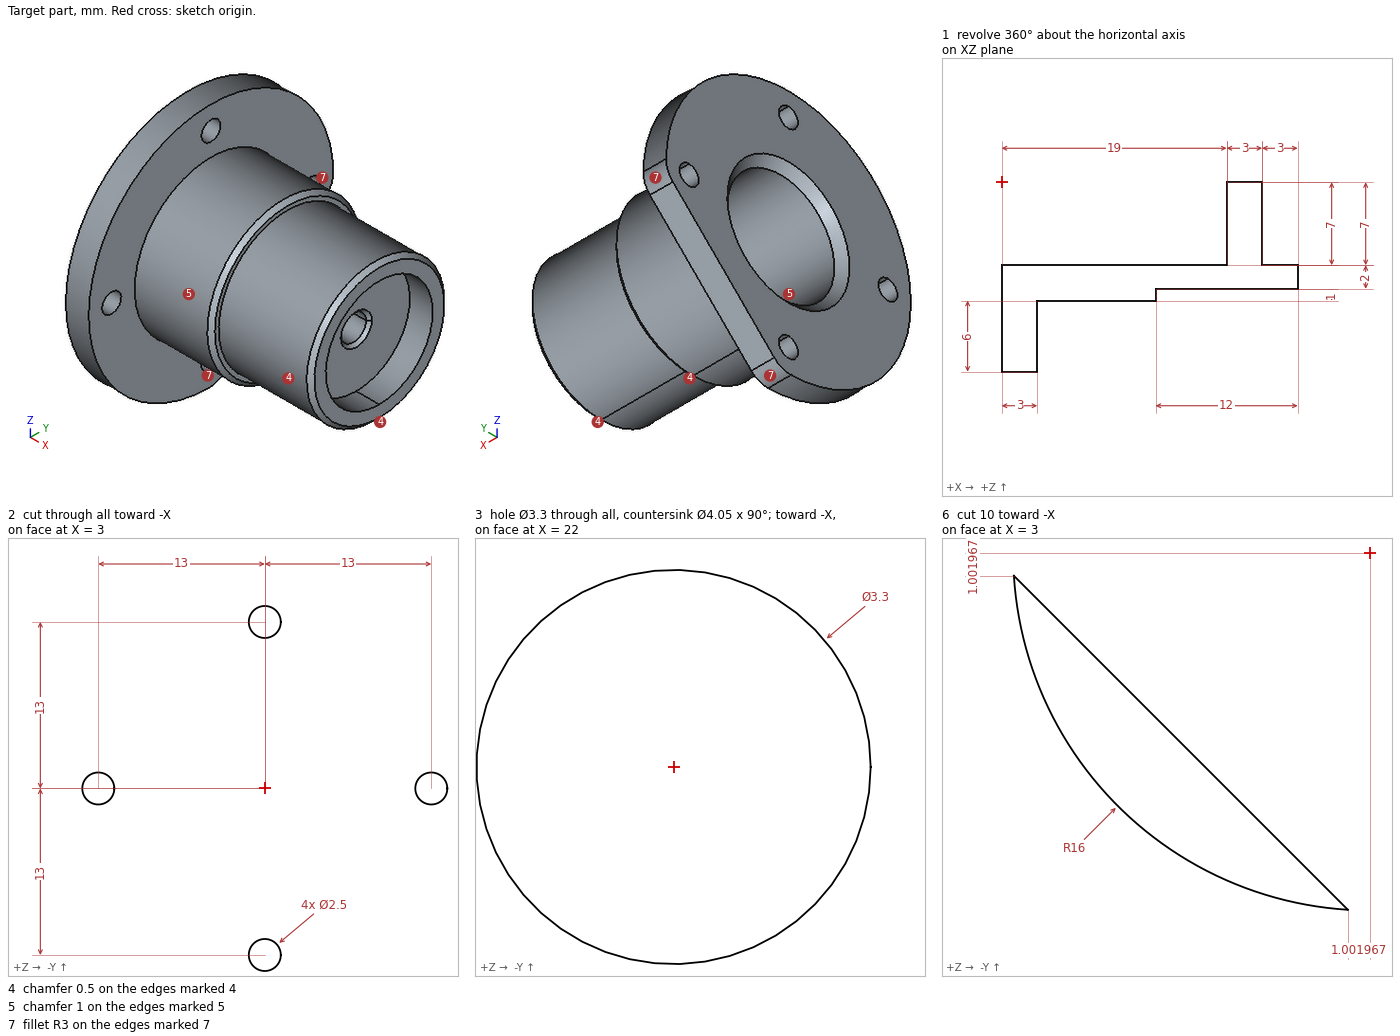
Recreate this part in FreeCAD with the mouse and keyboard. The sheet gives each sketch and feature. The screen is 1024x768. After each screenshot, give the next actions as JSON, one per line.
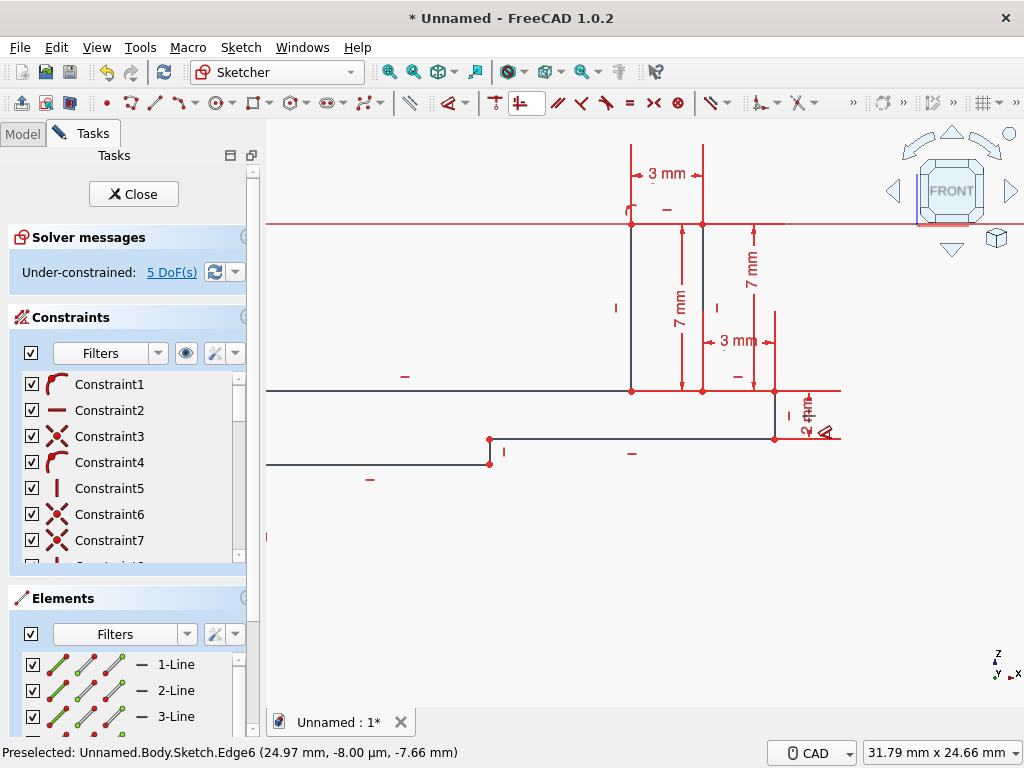
{"action": "scroll", "coordinate": [490, 449], "scroll_direction": "up", "scroll_amount": 3}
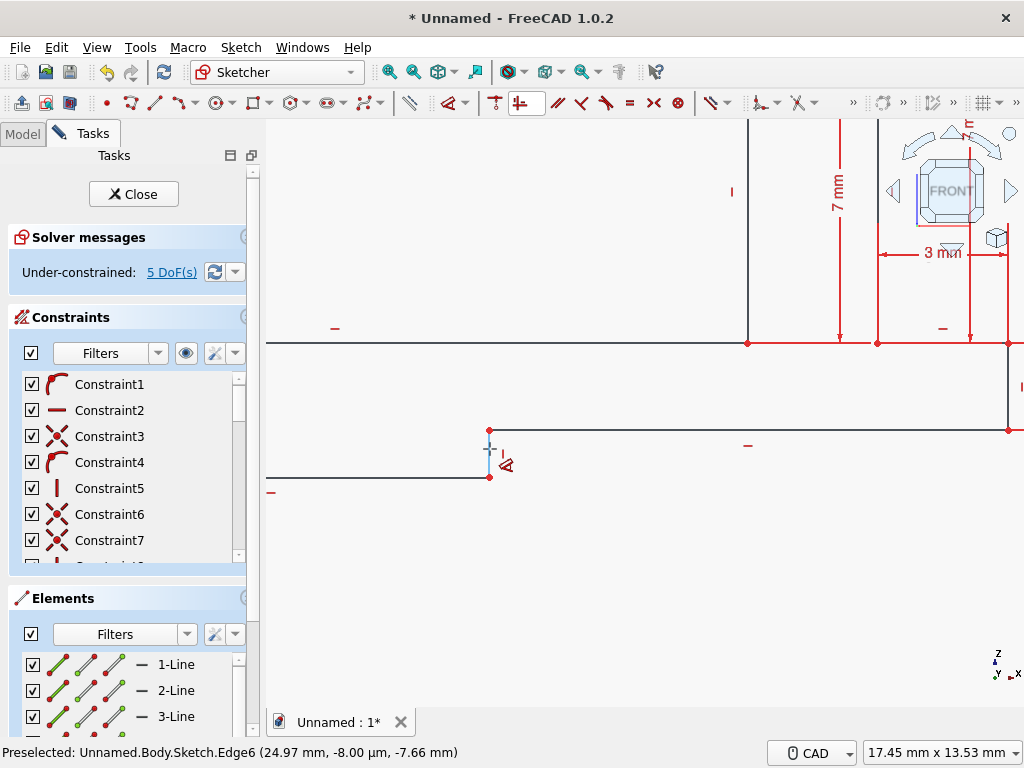
{"action": "left_click", "coordinate": [489, 449]}
{"action": "left_click", "coordinate": [523, 454]}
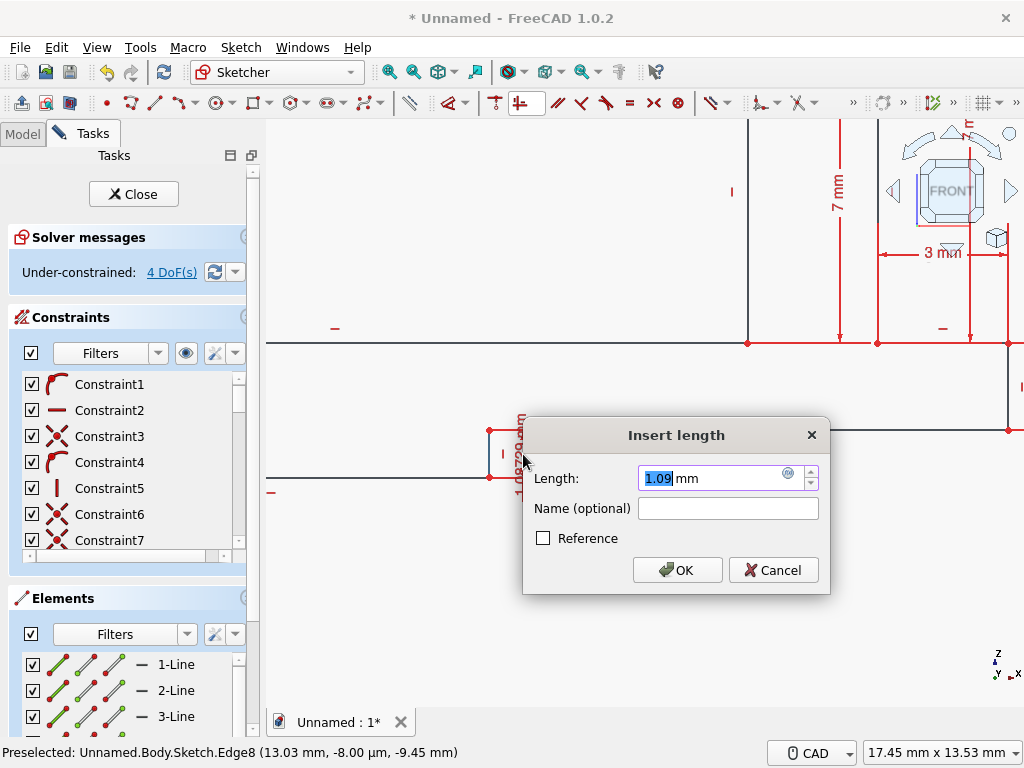
{"action": "type", "text": "1"}
{"action": "key", "text": "Return"}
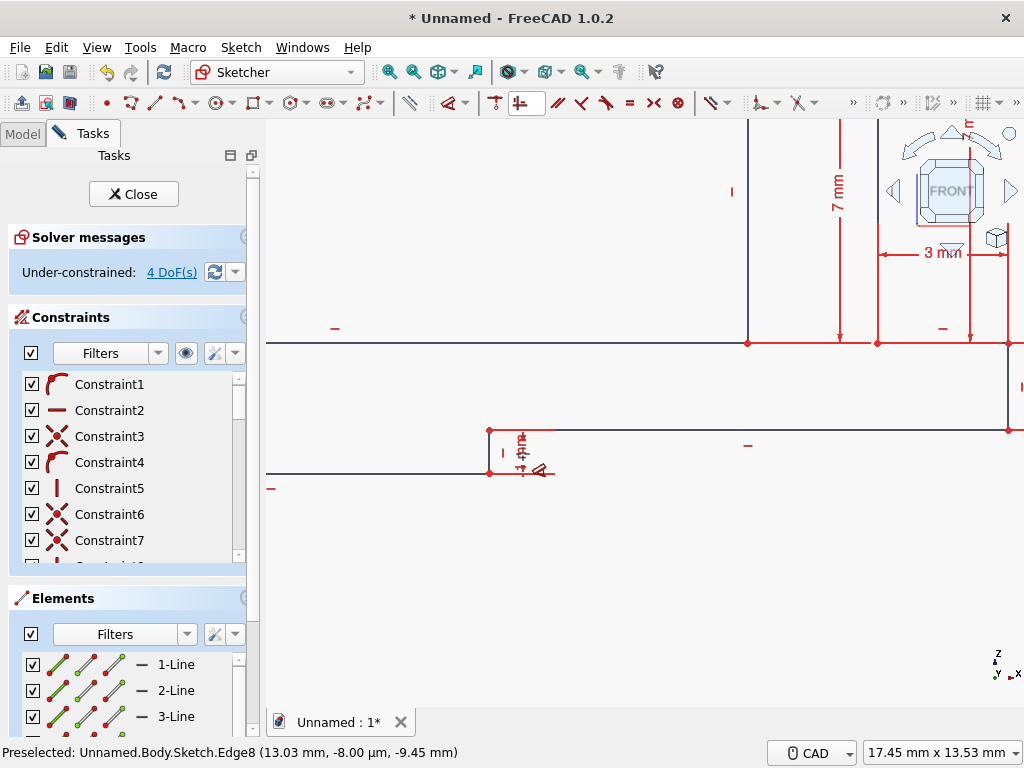
{"action": "scroll", "coordinate": [641, 428], "scroll_direction": "down", "scroll_amount": 5}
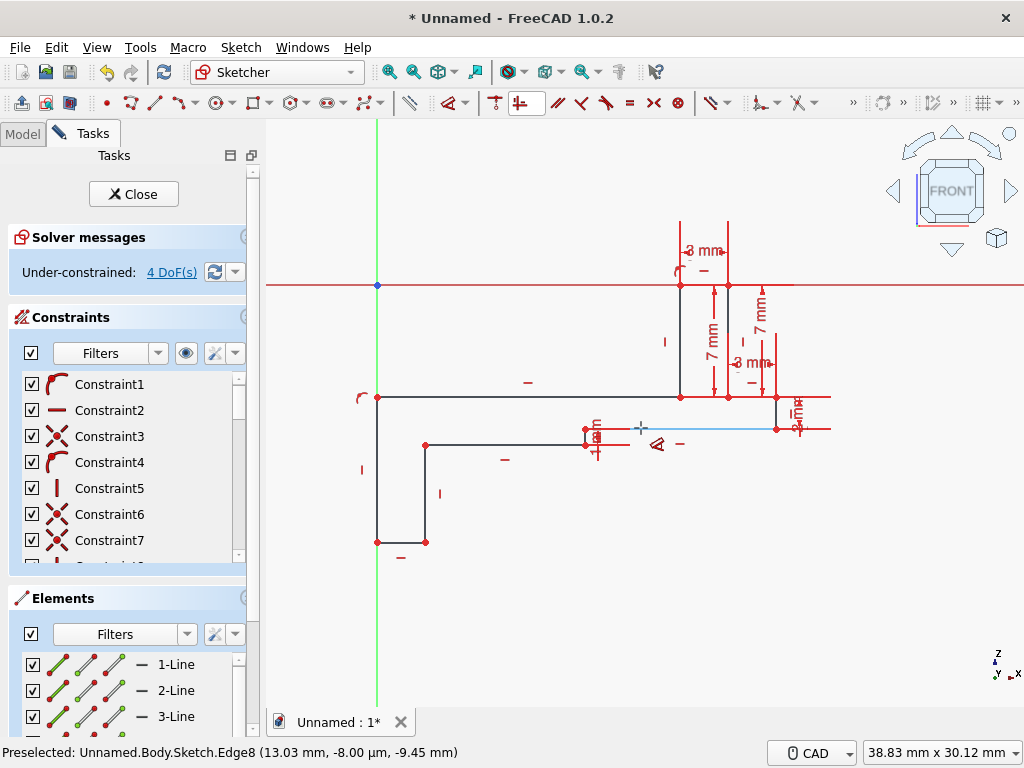
{"action": "left_click", "coordinate": [425, 474]}
{"action": "left_click", "coordinate": [391, 494]}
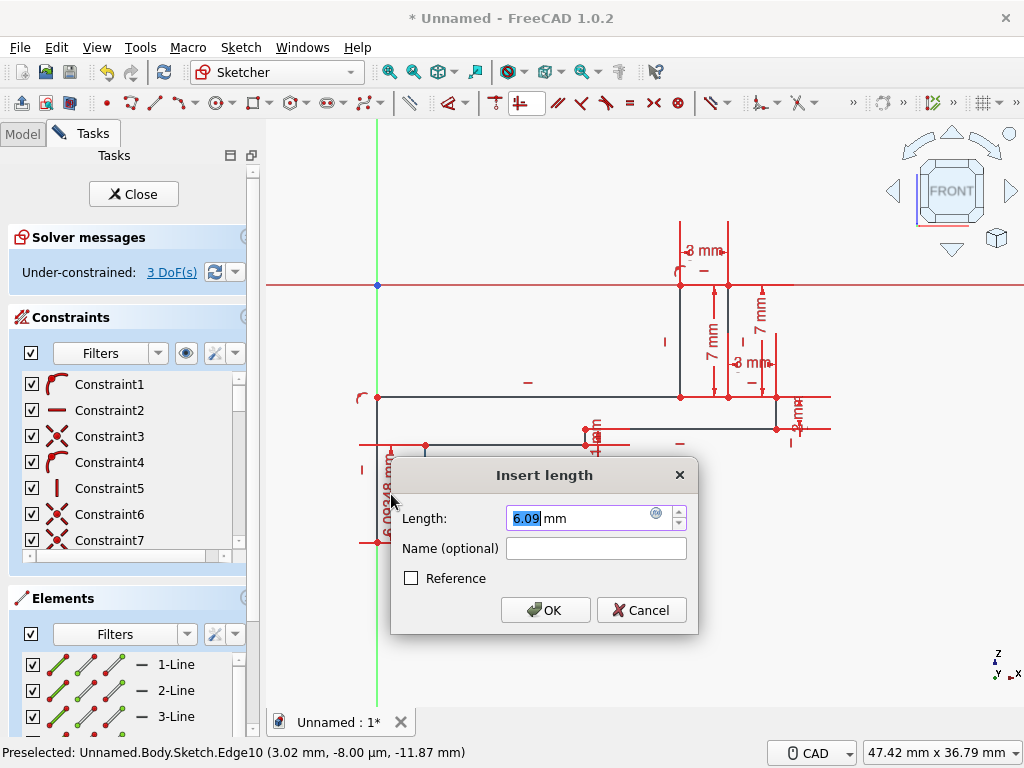
{"action": "type", "text": "6"}
{"action": "key", "text": "Return"}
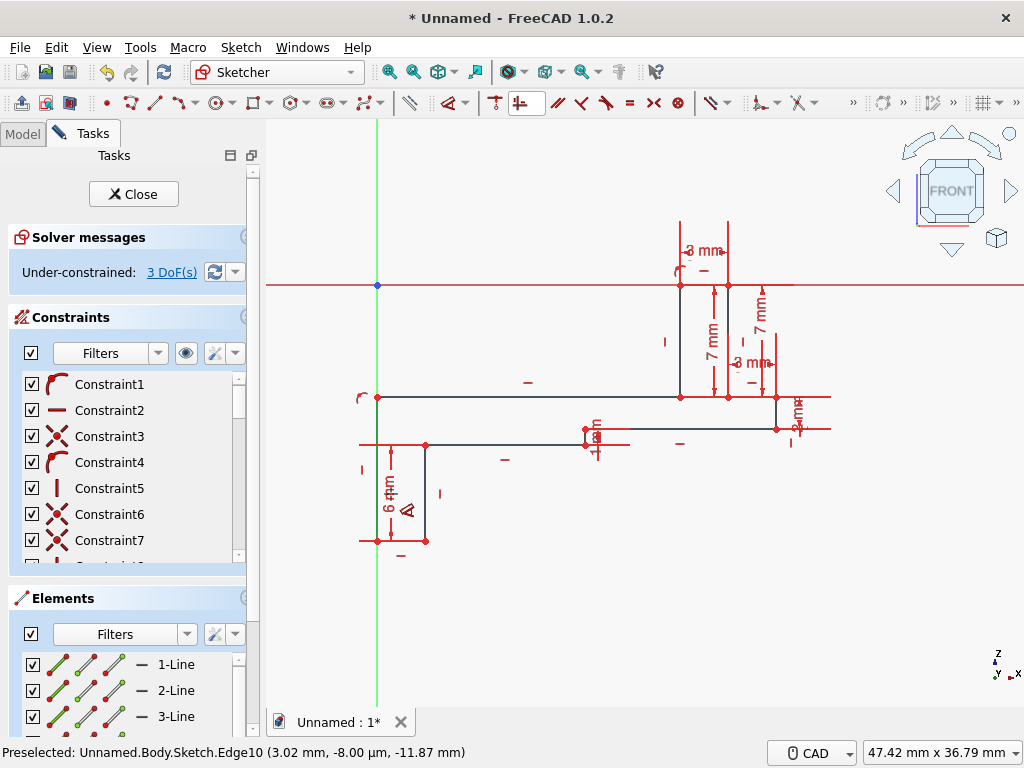
{"action": "left_click", "coordinate": [411, 541]}
{"action": "left_click", "coordinate": [401, 575]}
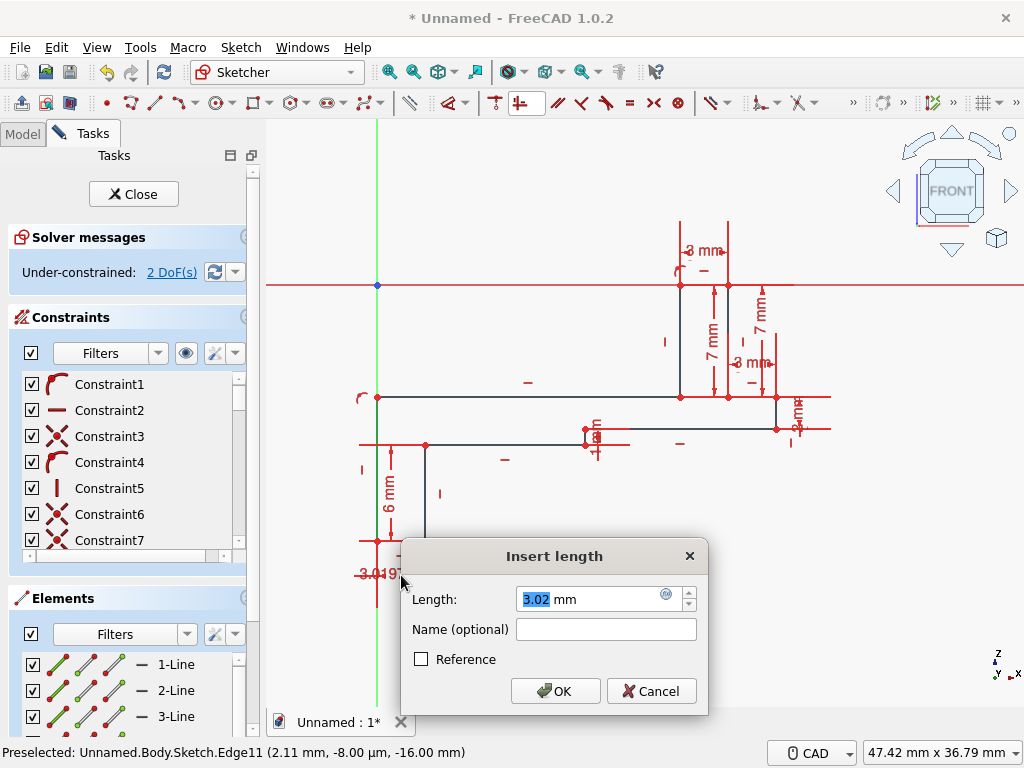
{"action": "type", "text": "3"}
{"action": "key", "text": "Return"}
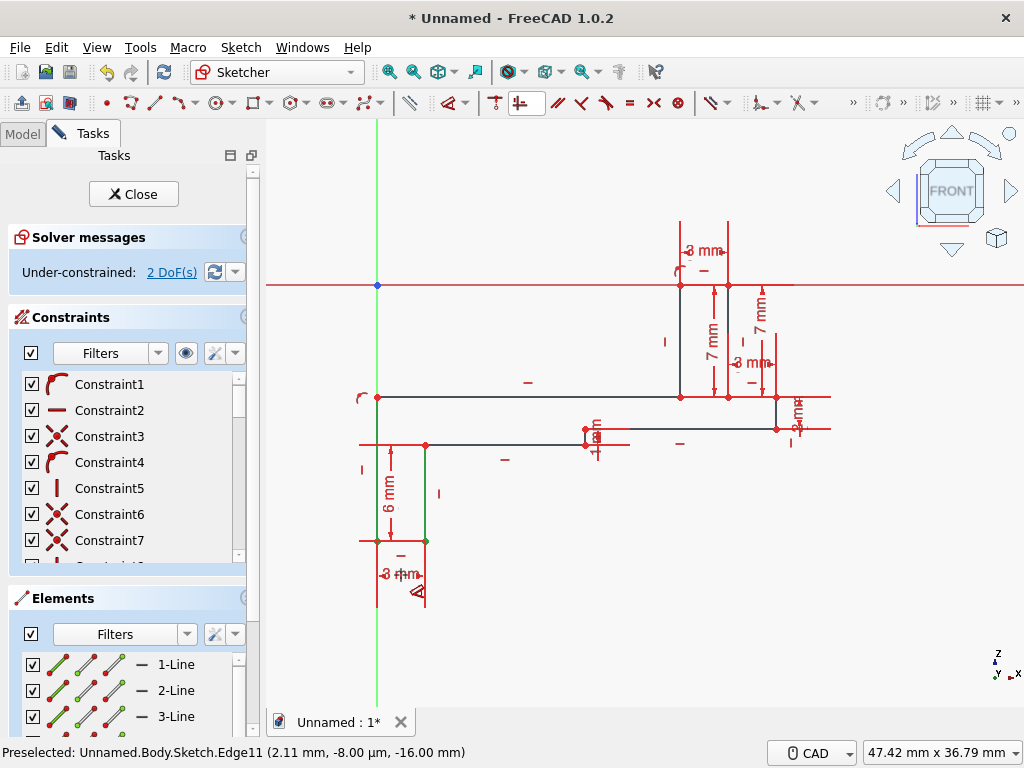
{"action": "left_click", "coordinate": [468, 397]}
{"action": "left_click", "coordinate": [529, 363]}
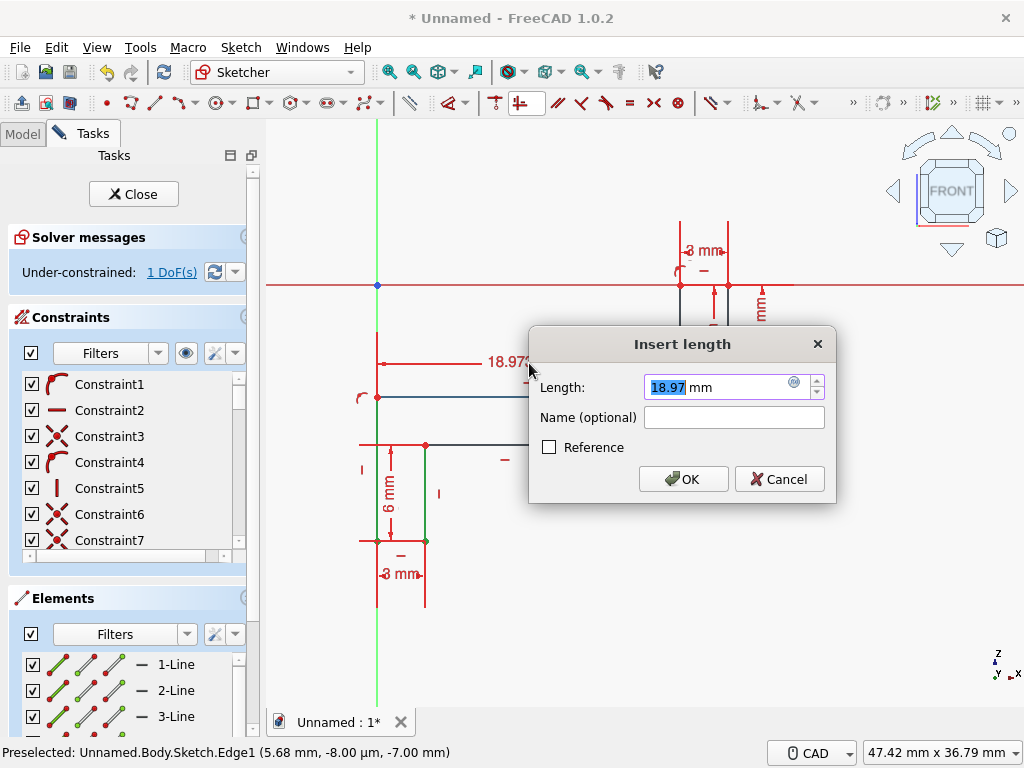
{"action": "type", "text": "19"}
{"action": "key", "text": "Return"}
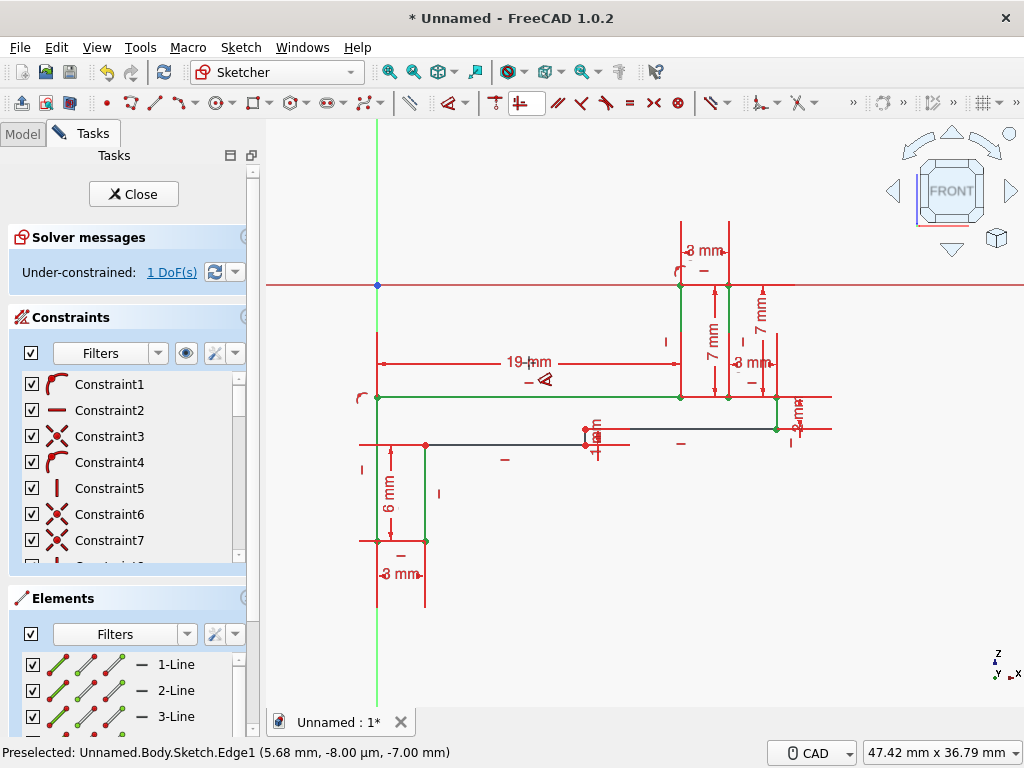
{"action": "left_click", "coordinate": [719, 429]}
{"action": "left_click", "coordinate": [681, 463]}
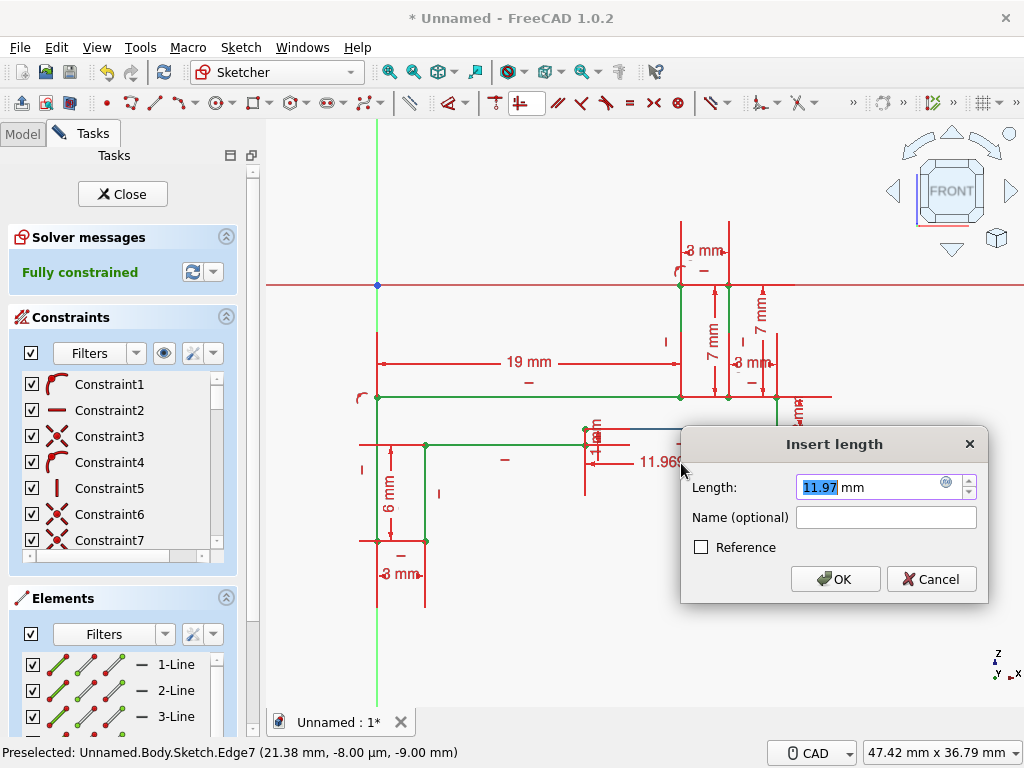
{"action": "type", "text": "12"}
{"action": "key", "text": "Return"}
{"action": "key", "text": "Escape"}